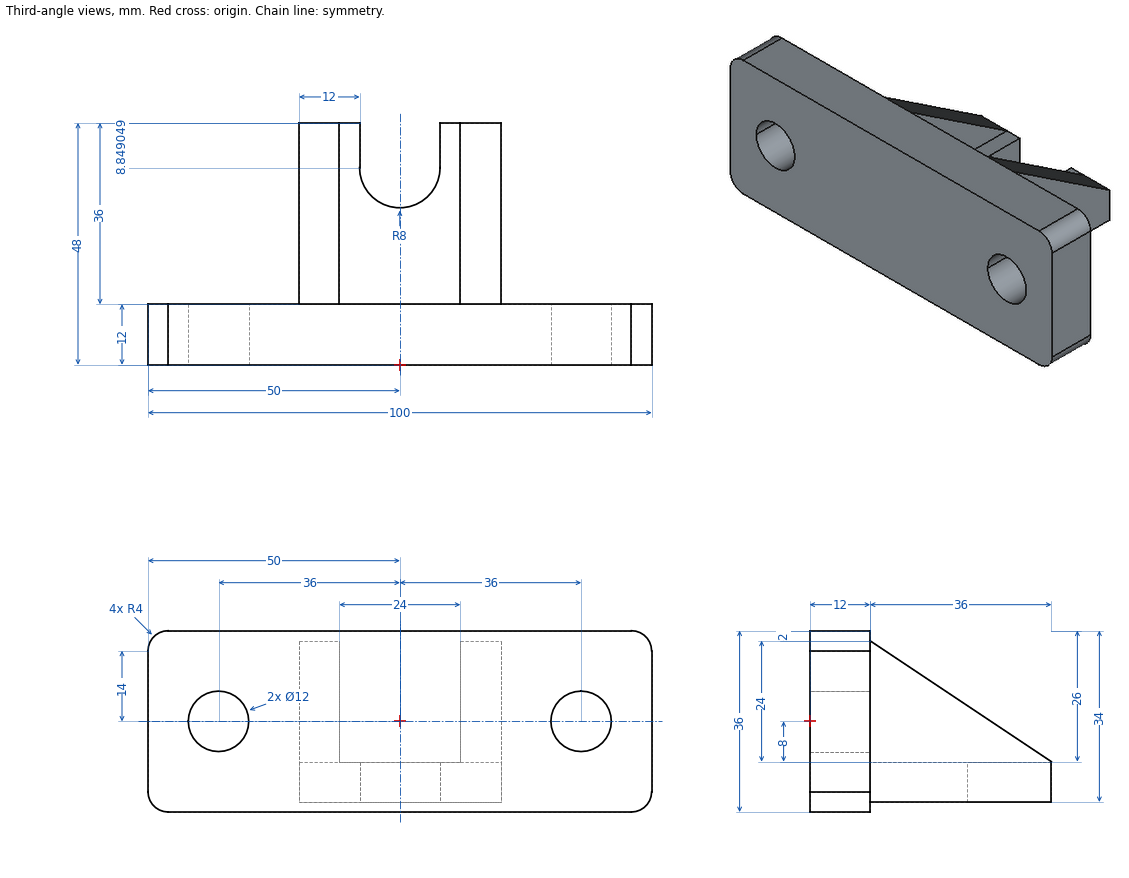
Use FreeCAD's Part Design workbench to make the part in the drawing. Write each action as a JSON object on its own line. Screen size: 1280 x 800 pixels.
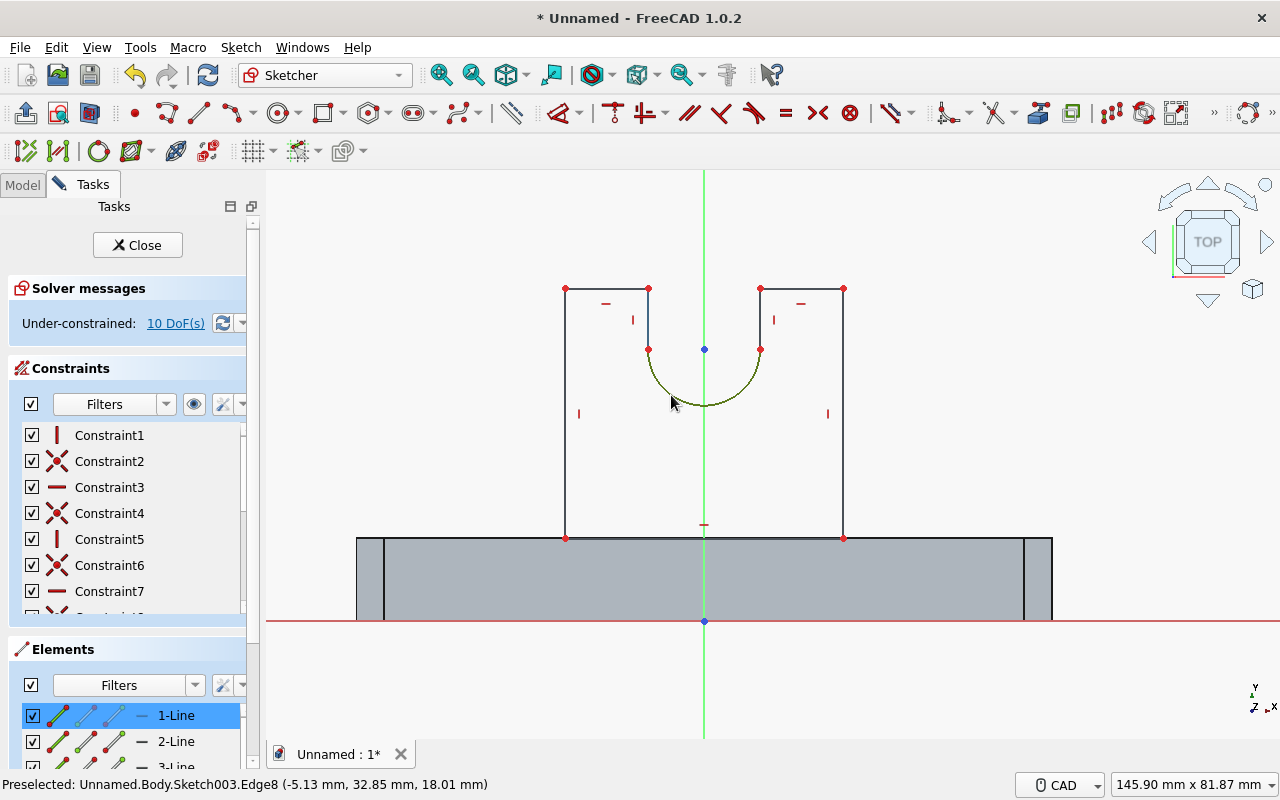
{"action": "left_click", "coordinate": [754, 114]}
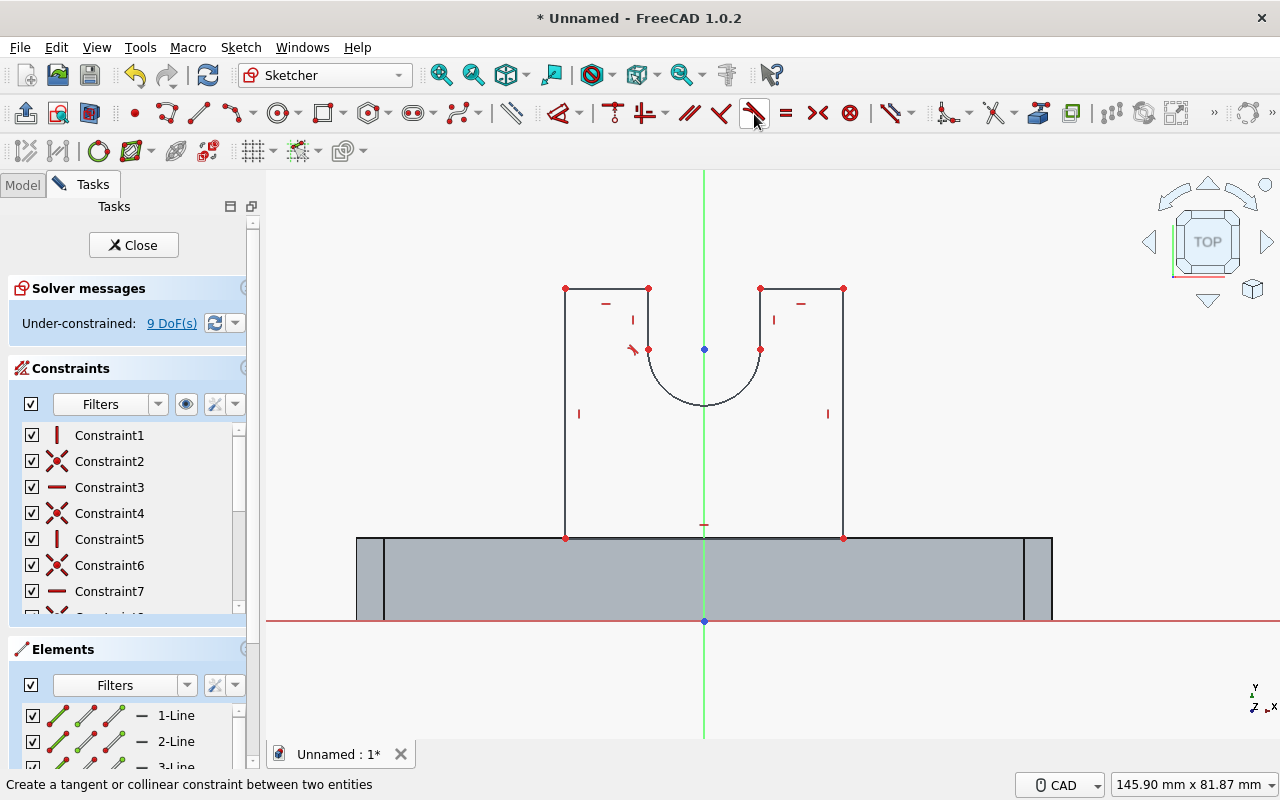
{"action": "left_click", "coordinate": [760, 307]}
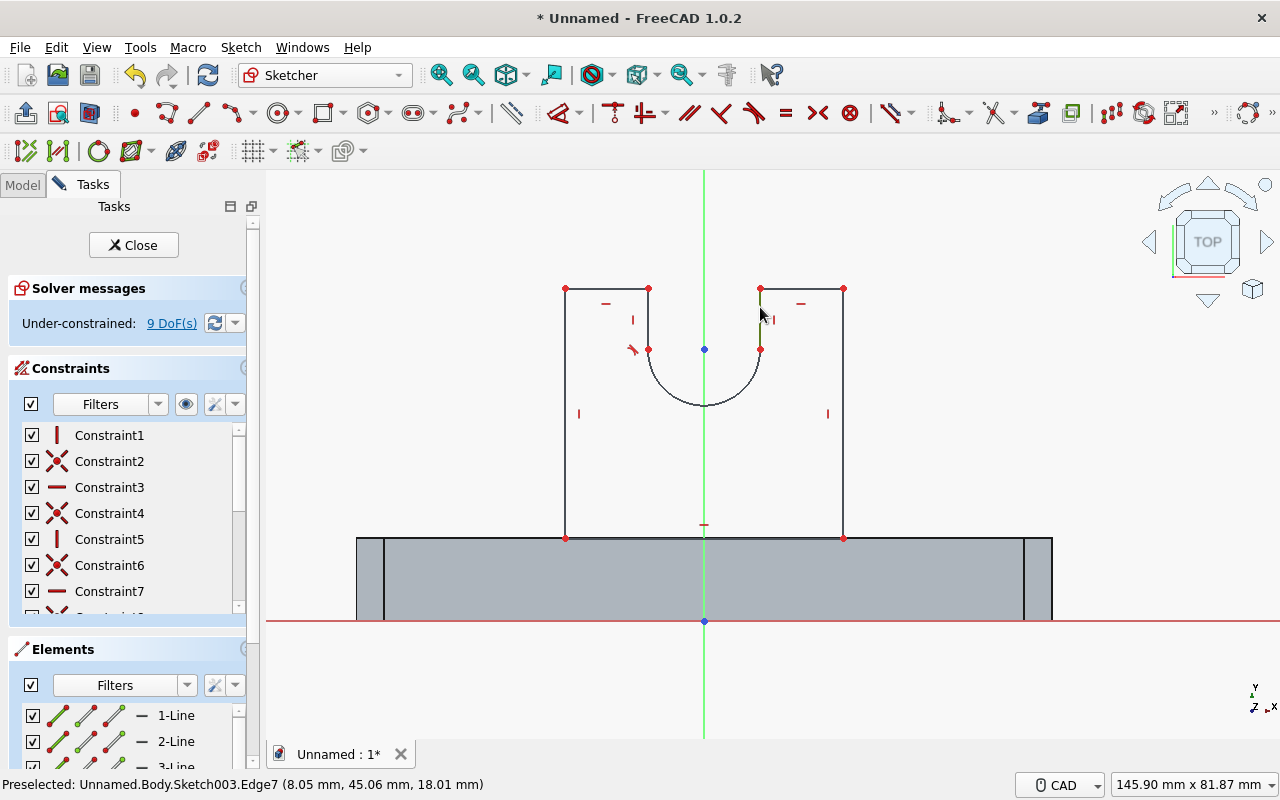
{"action": "left_click", "coordinate": [671, 395]}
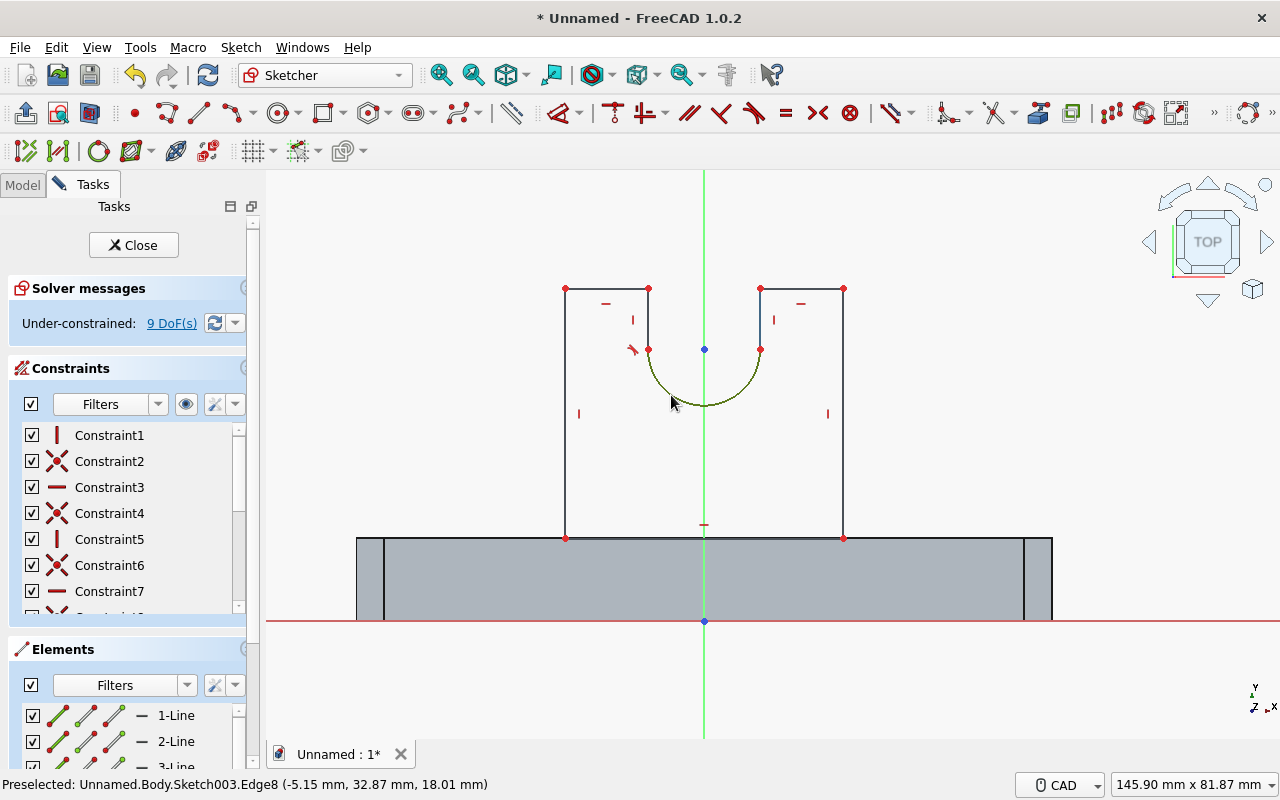
{"action": "left_click", "coordinate": [754, 114]}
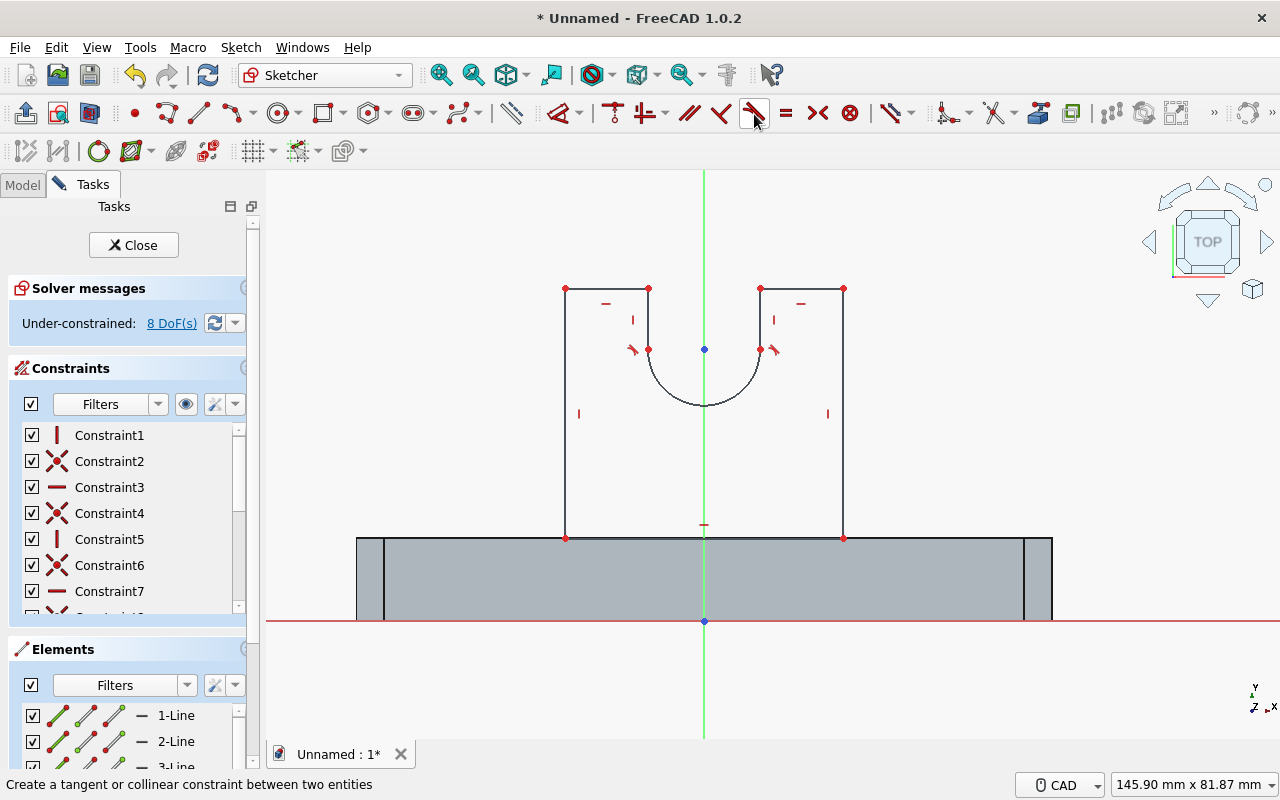
{"action": "left_click", "coordinate": [704, 350]}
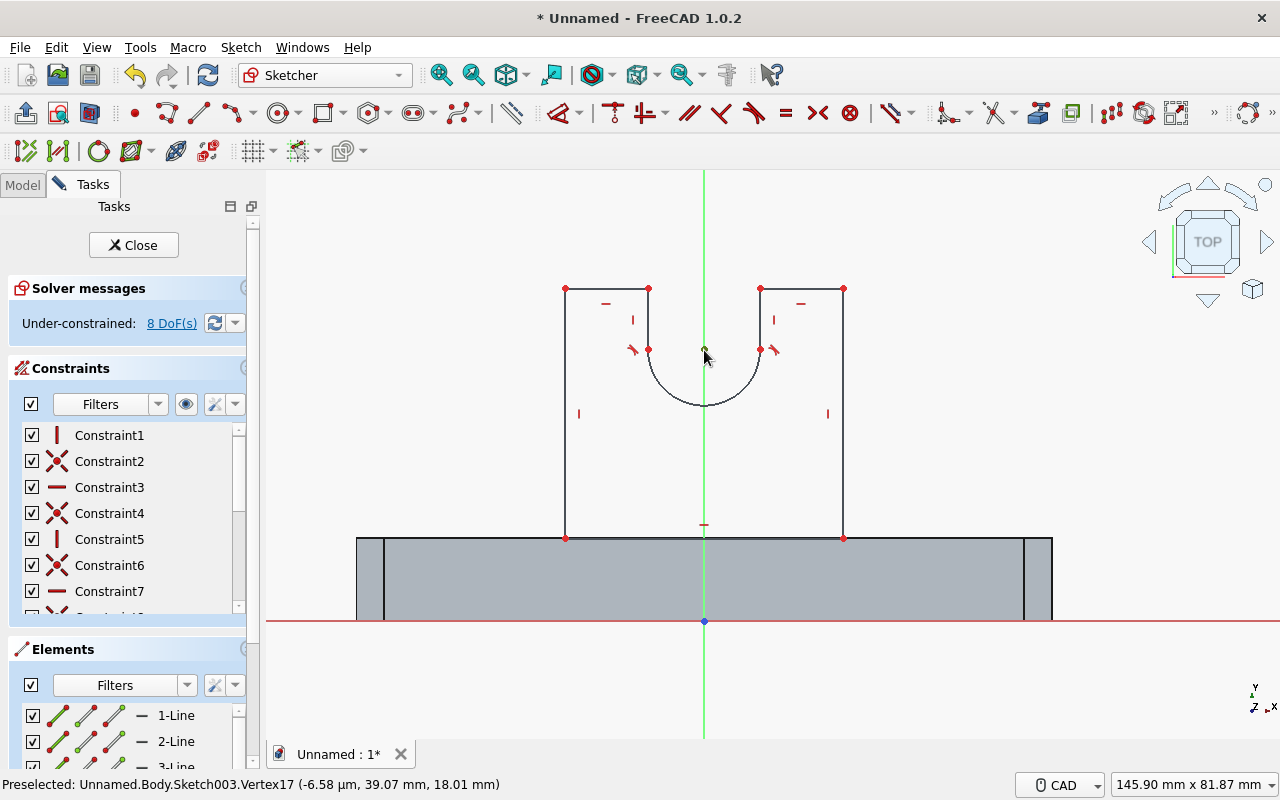
{"action": "left_click", "coordinate": [704, 674]}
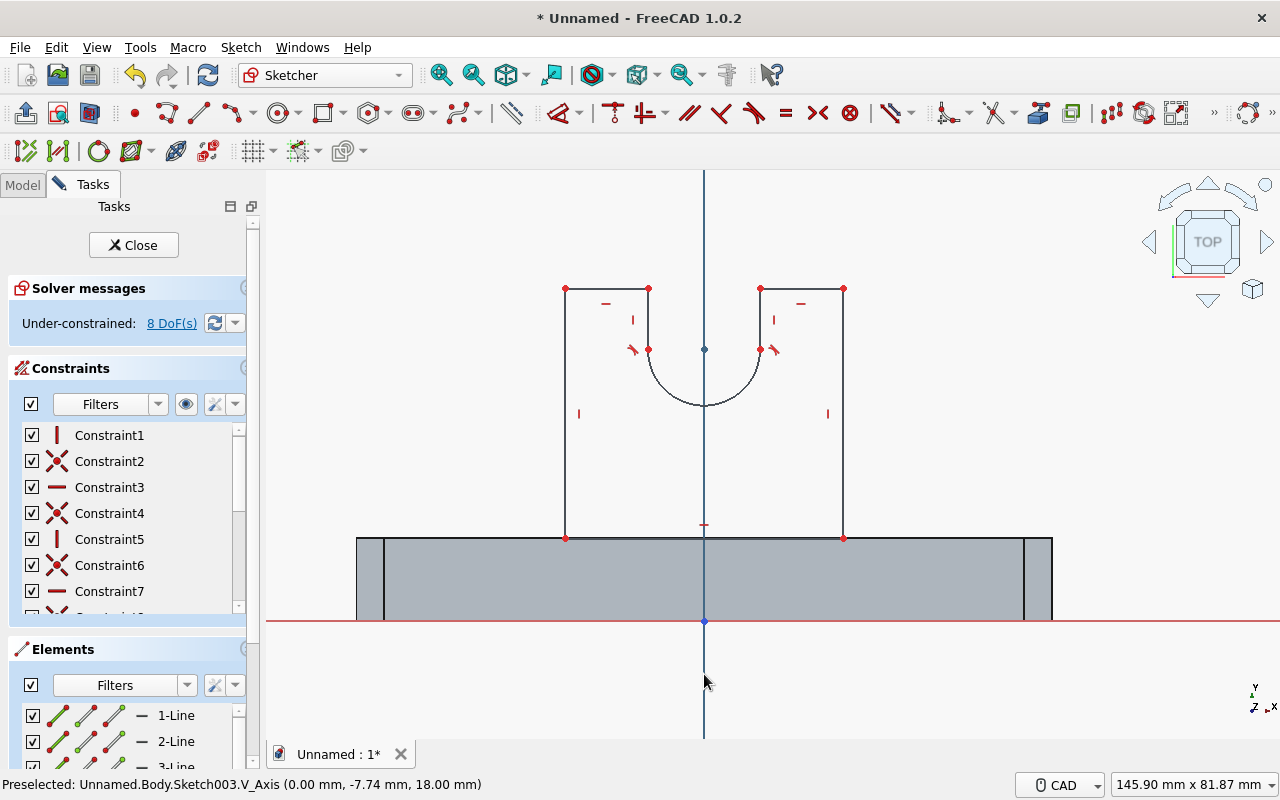
{"action": "left_click", "coordinate": [614, 114]}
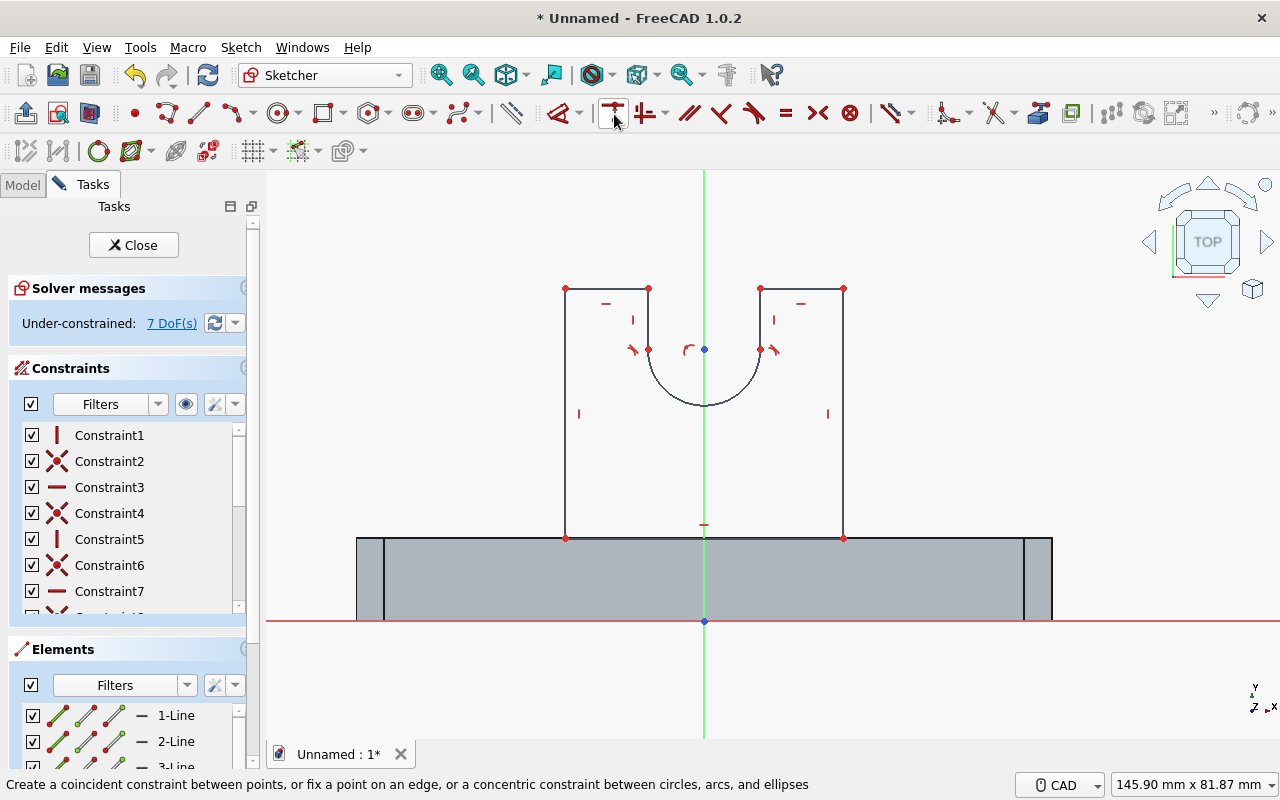
{"action": "left_click", "coordinate": [565, 289]}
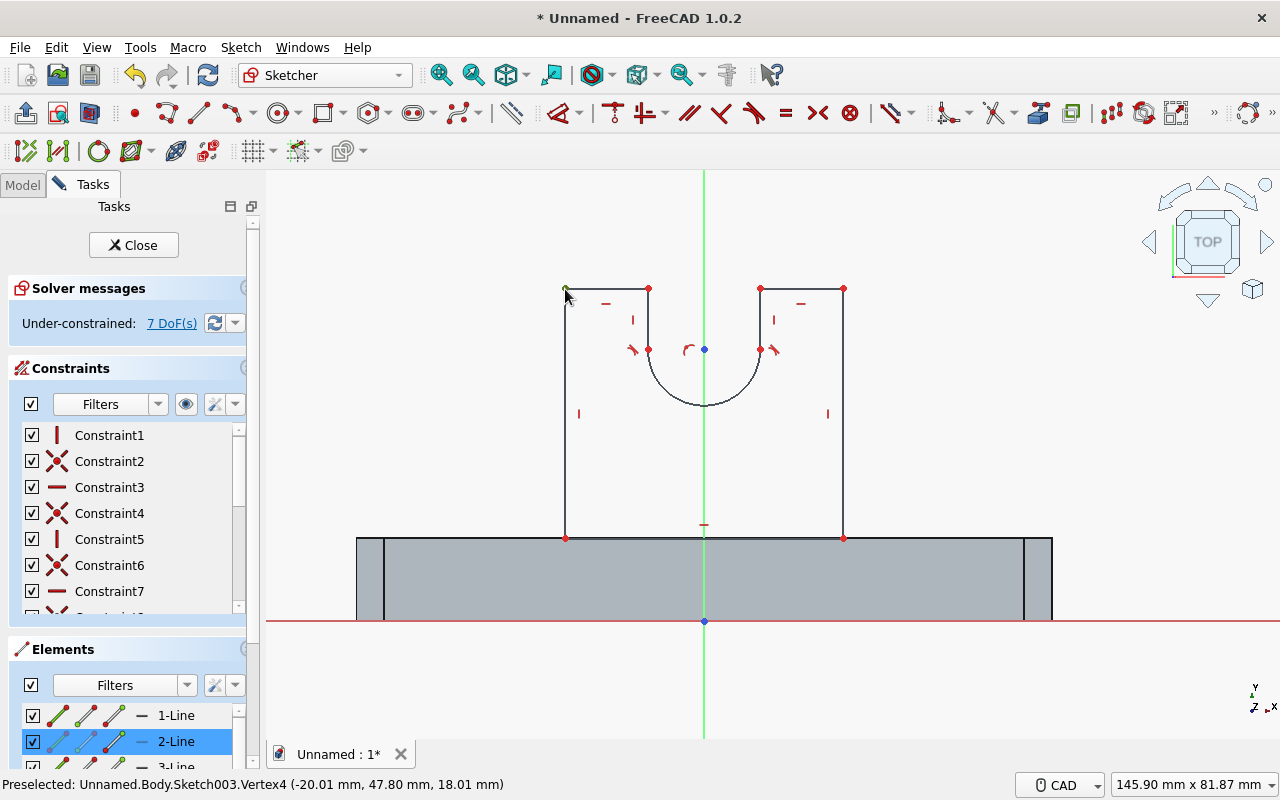
{"action": "left_click", "coordinate": [843, 289]}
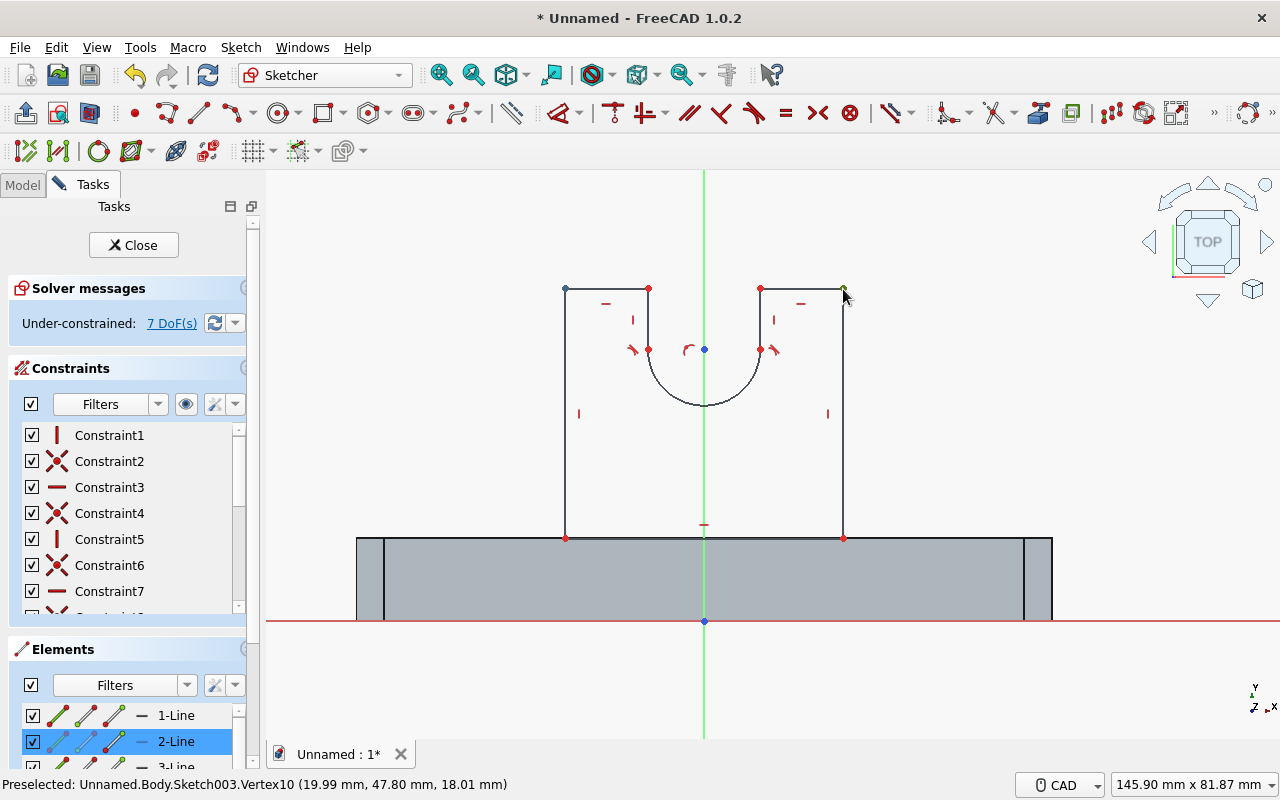
{"action": "left_click", "coordinate": [704, 674]}